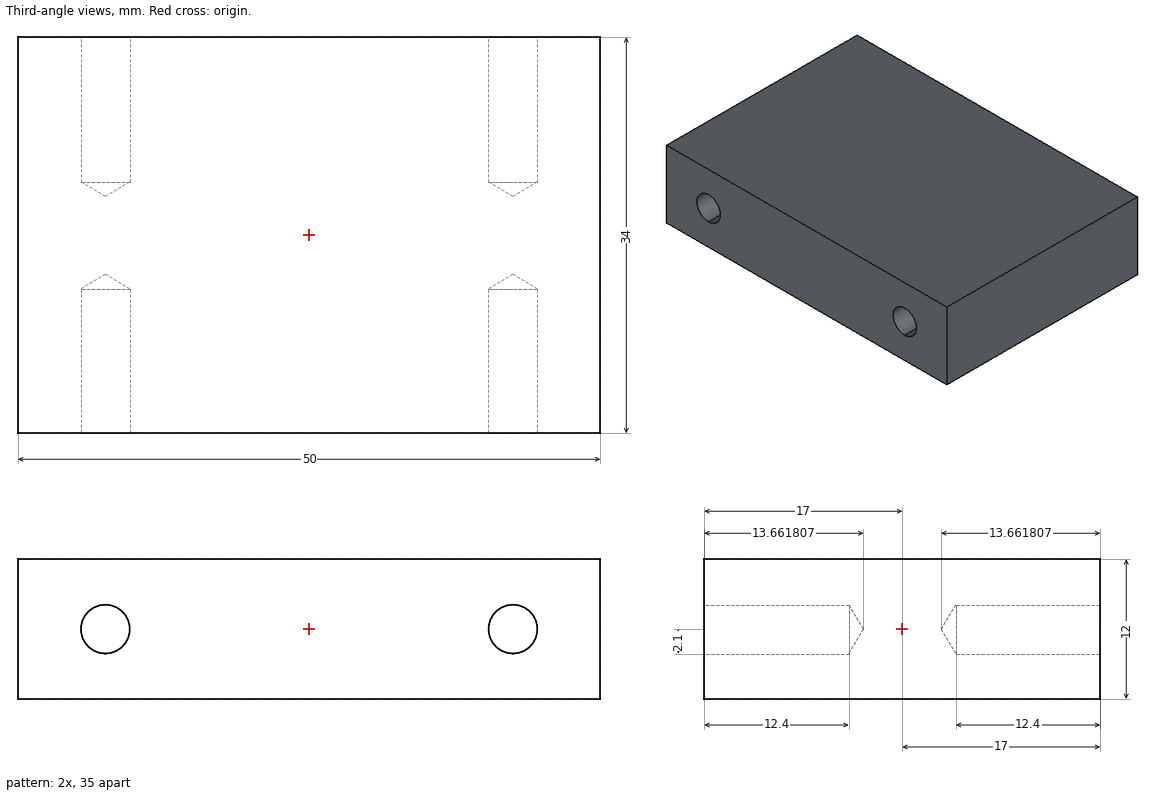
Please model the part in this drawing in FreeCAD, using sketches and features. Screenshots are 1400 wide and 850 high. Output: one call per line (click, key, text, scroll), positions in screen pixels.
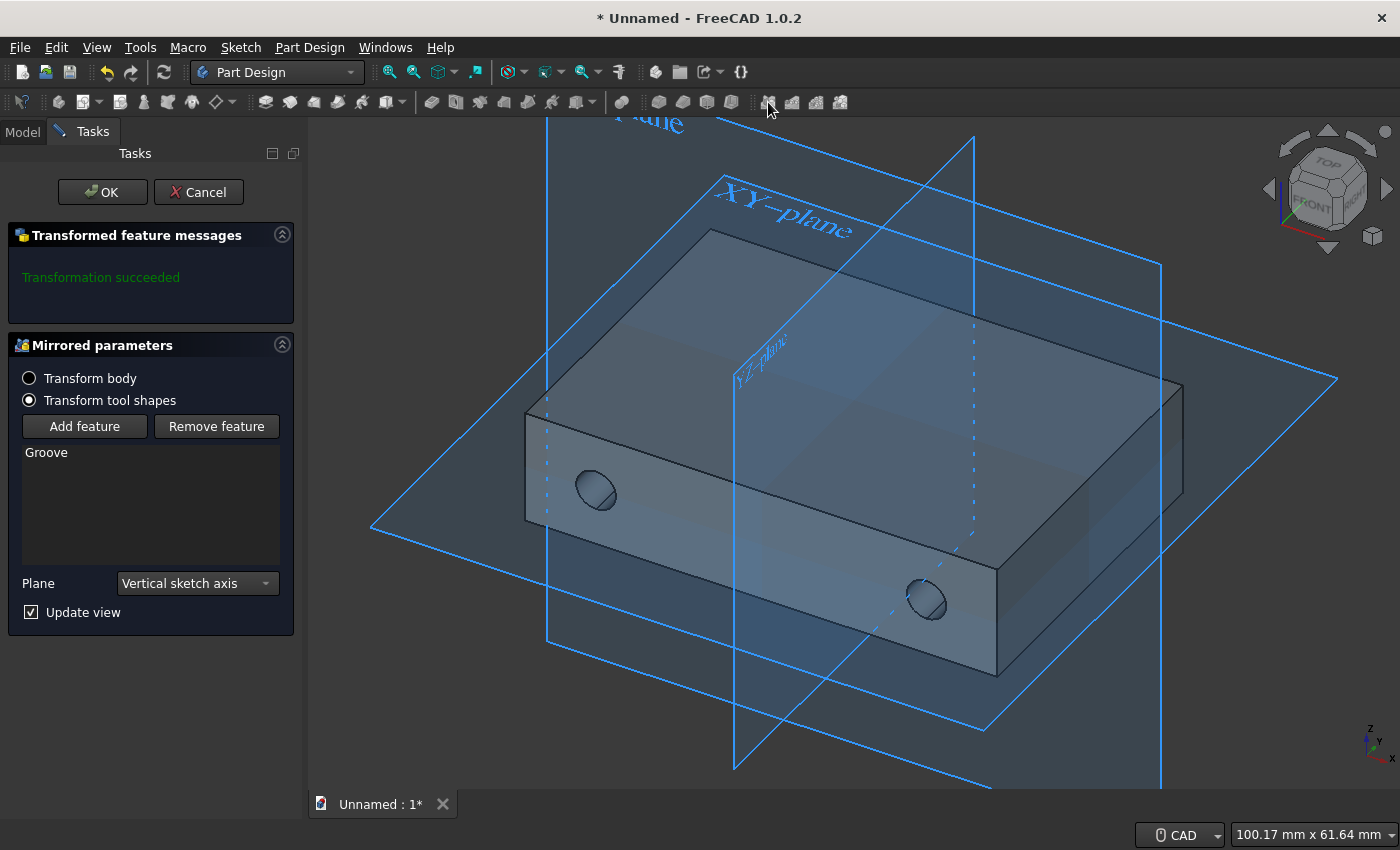
click(198, 584)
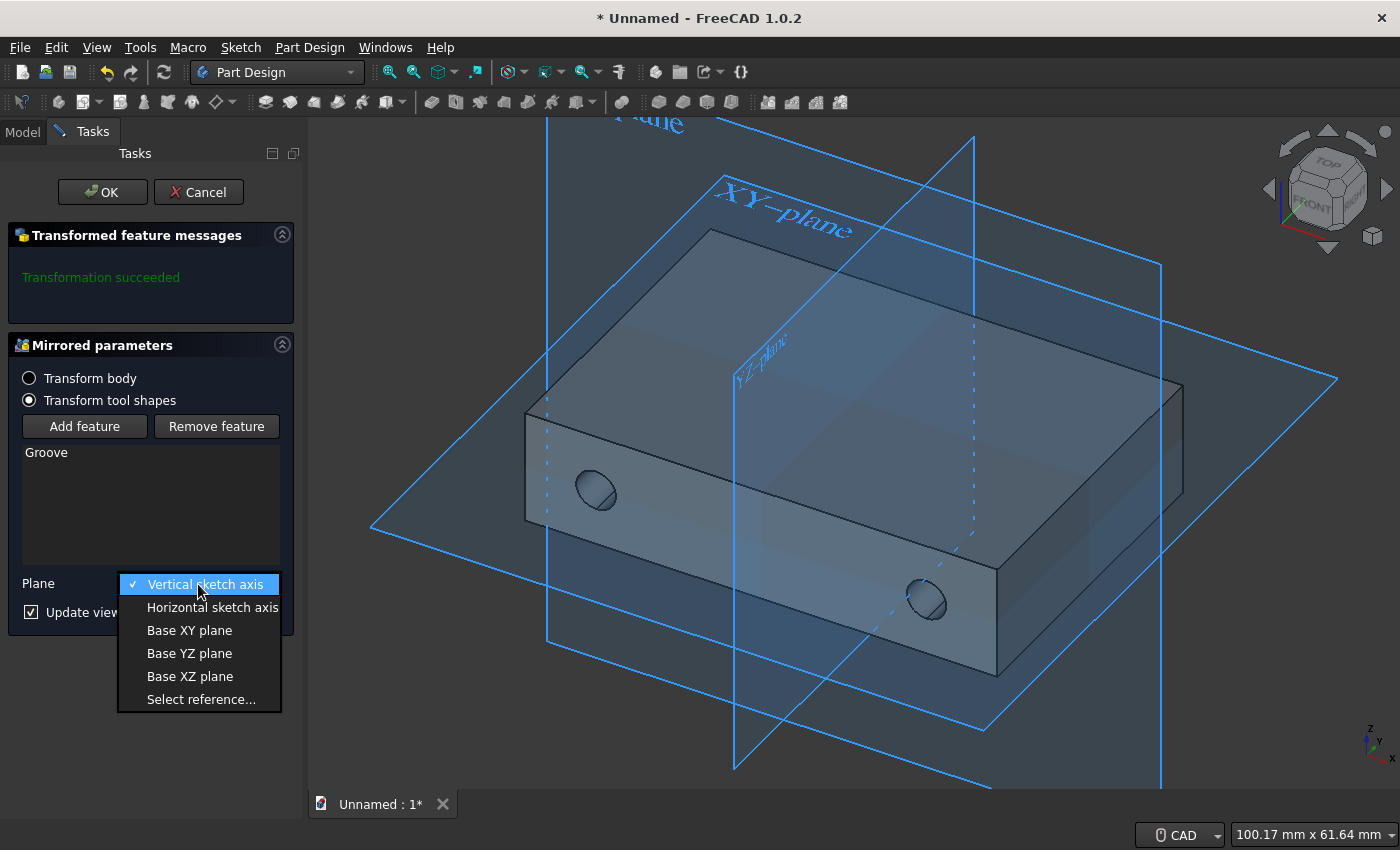
click(198, 676)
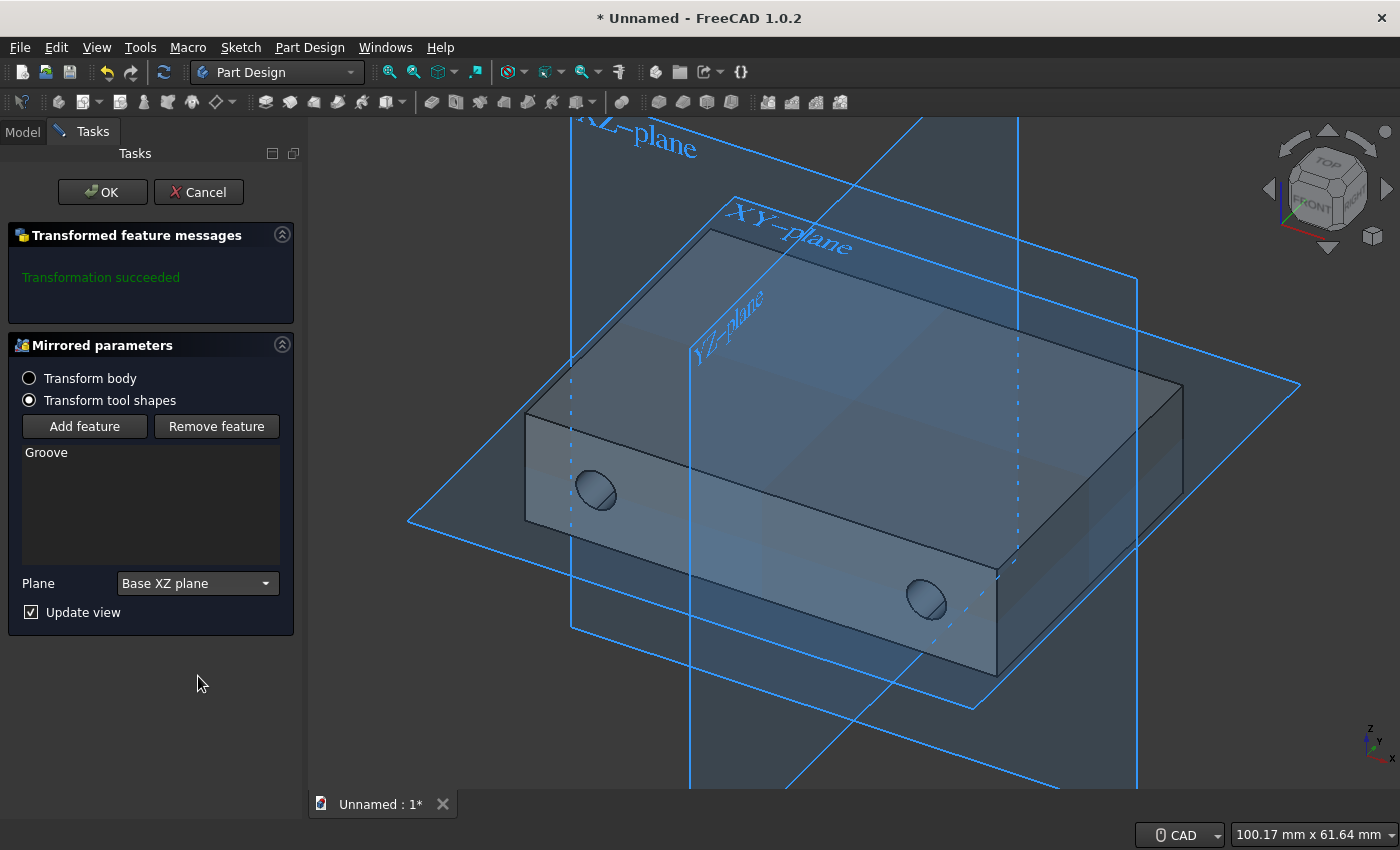
click(103, 192)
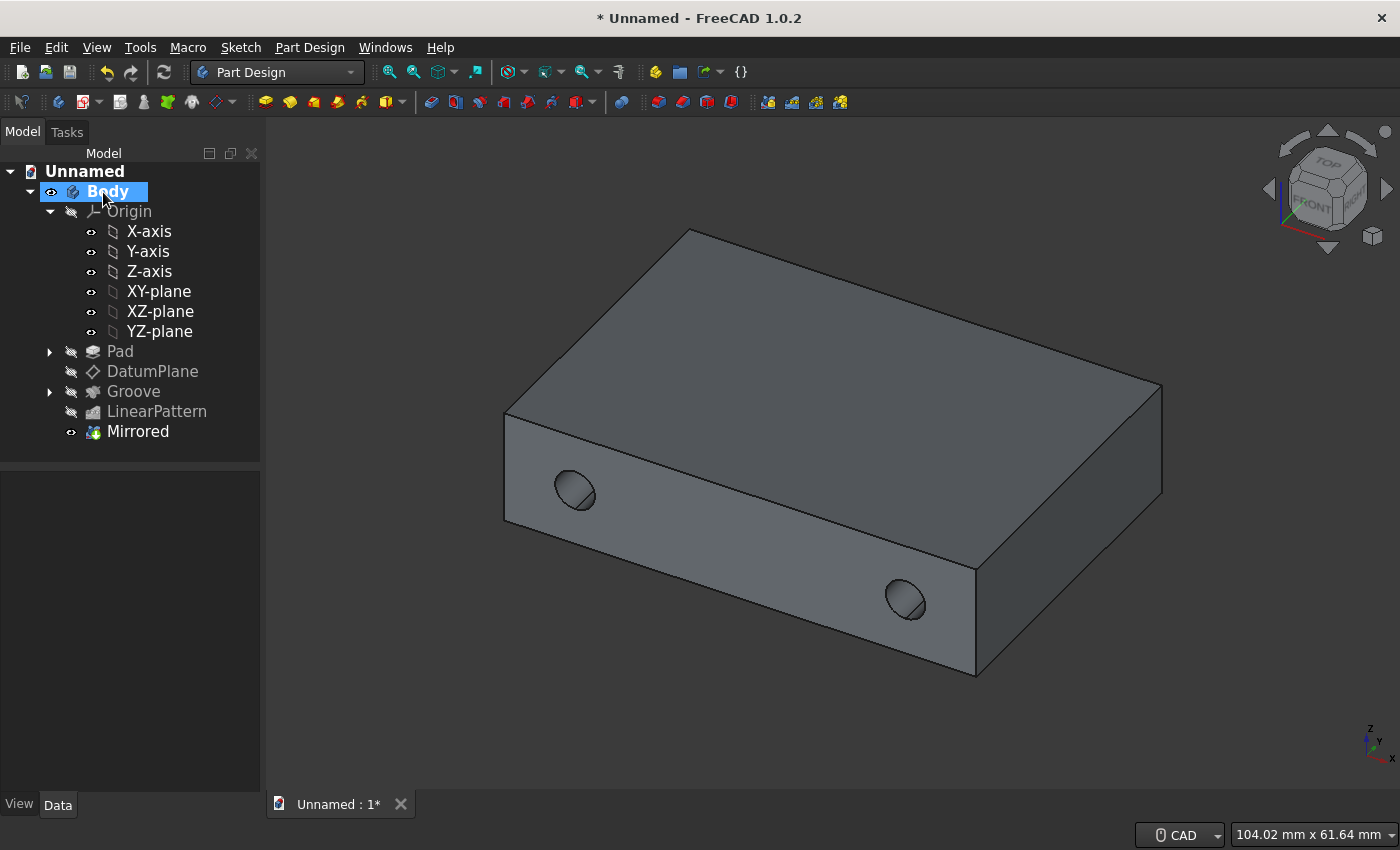
click(136, 332)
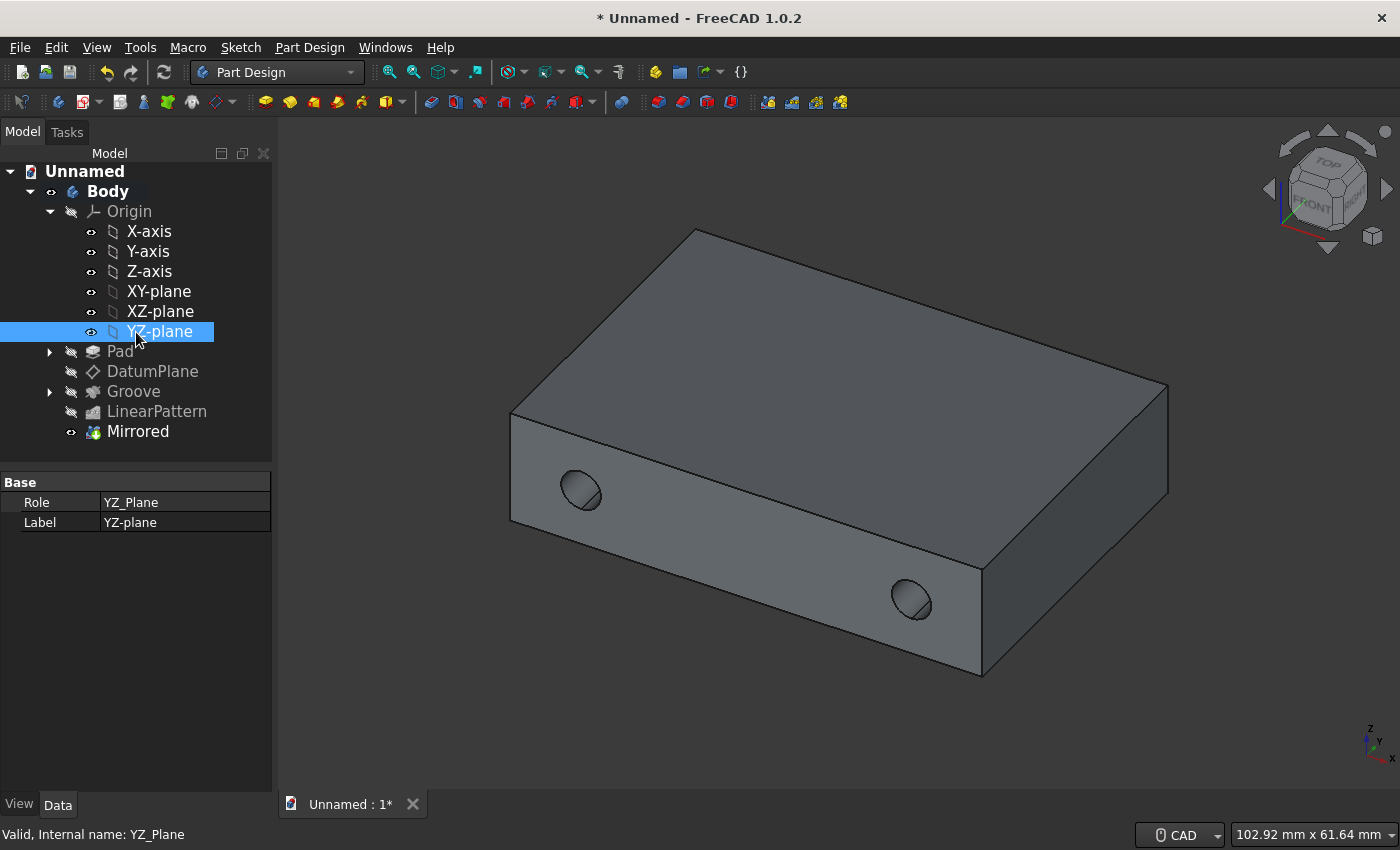
click(216, 102)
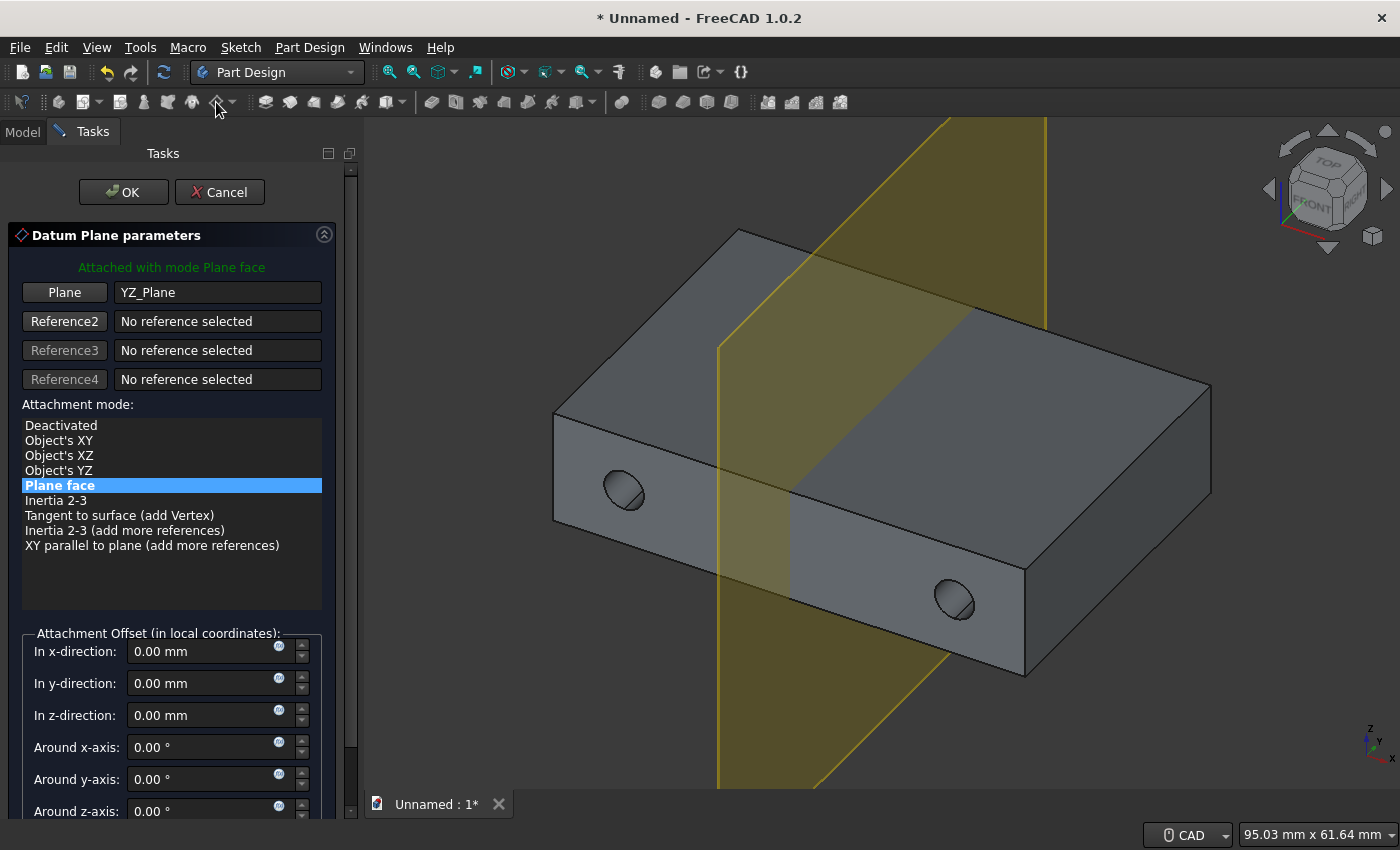
triple_click(210, 715)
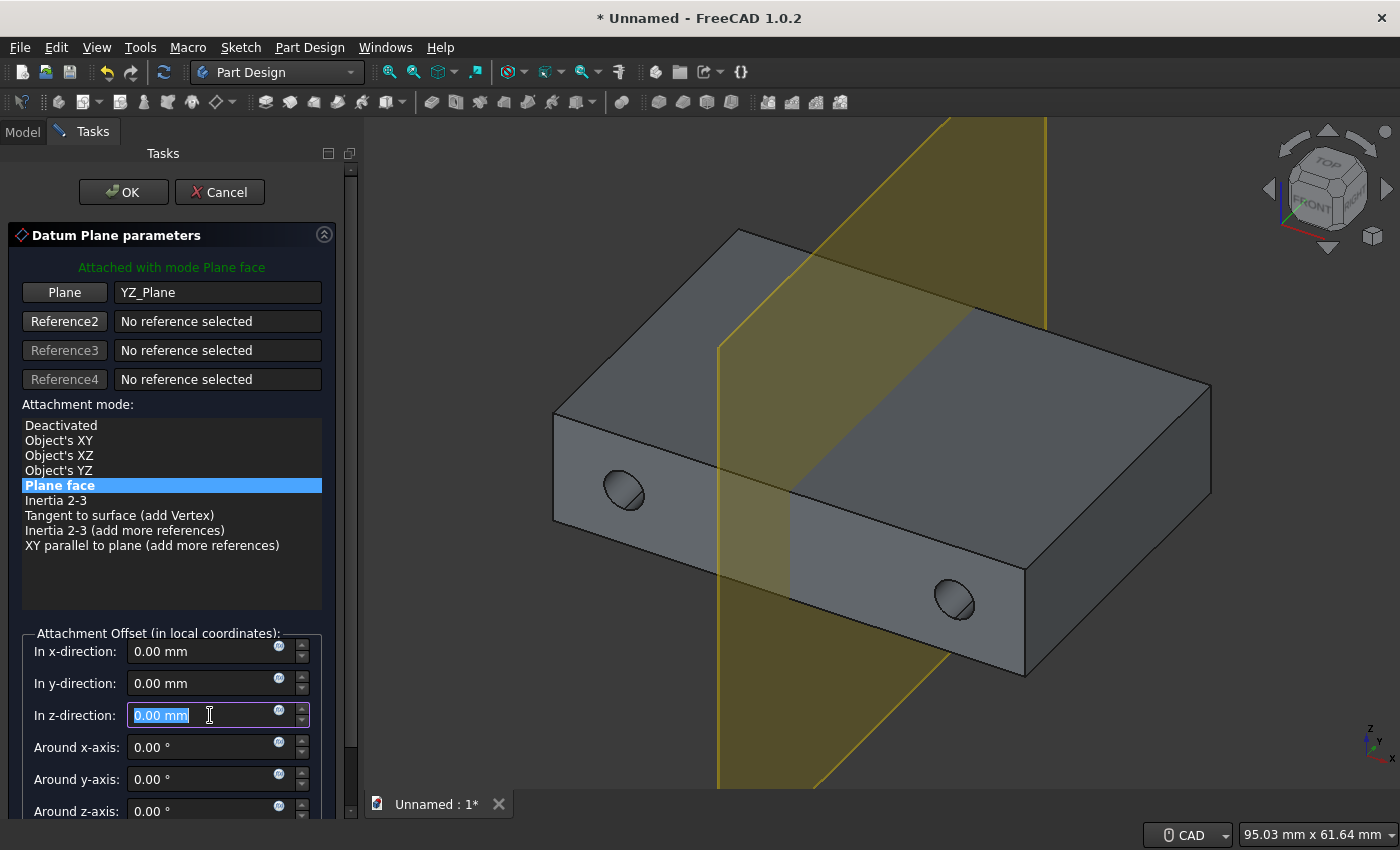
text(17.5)
key(Tab)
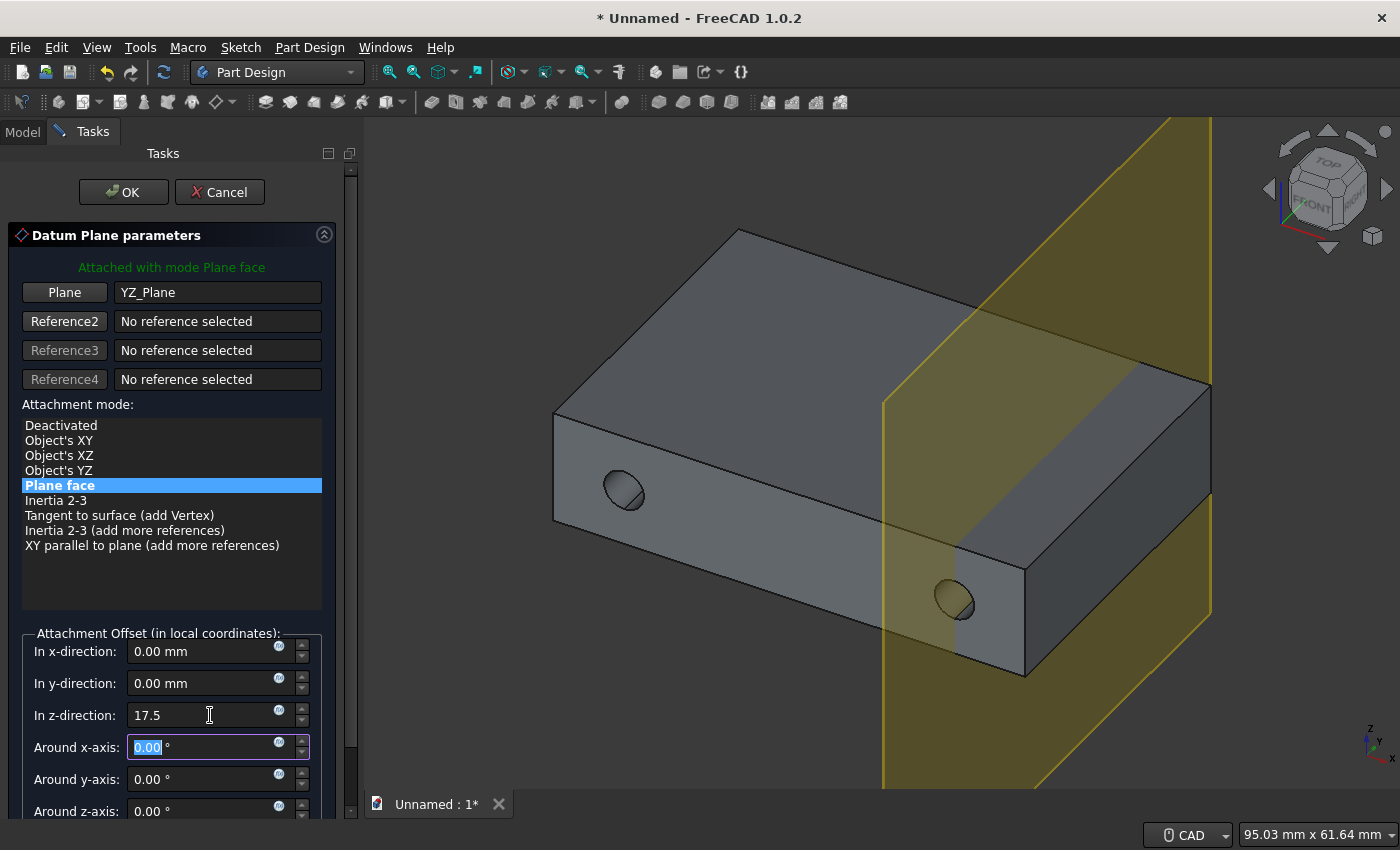
click(124, 192)